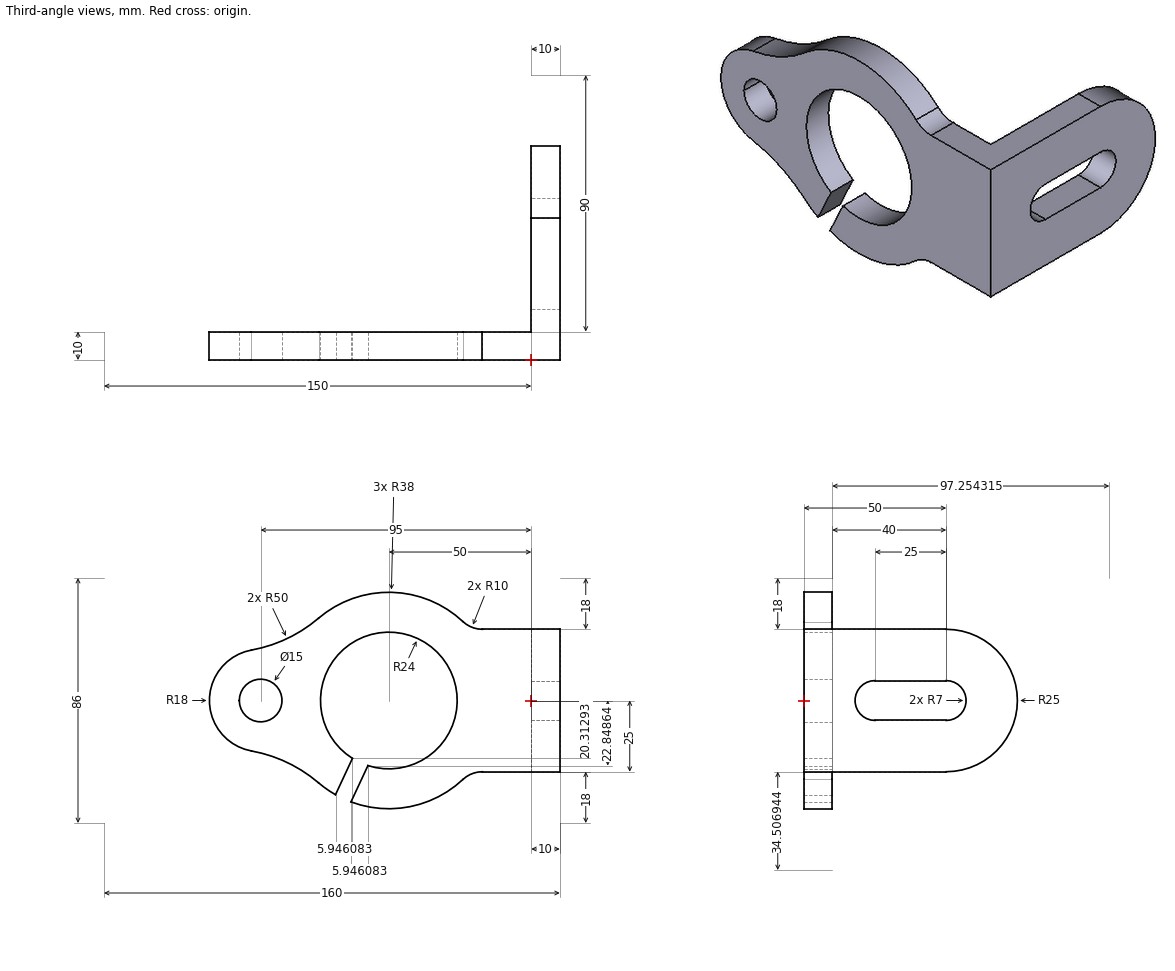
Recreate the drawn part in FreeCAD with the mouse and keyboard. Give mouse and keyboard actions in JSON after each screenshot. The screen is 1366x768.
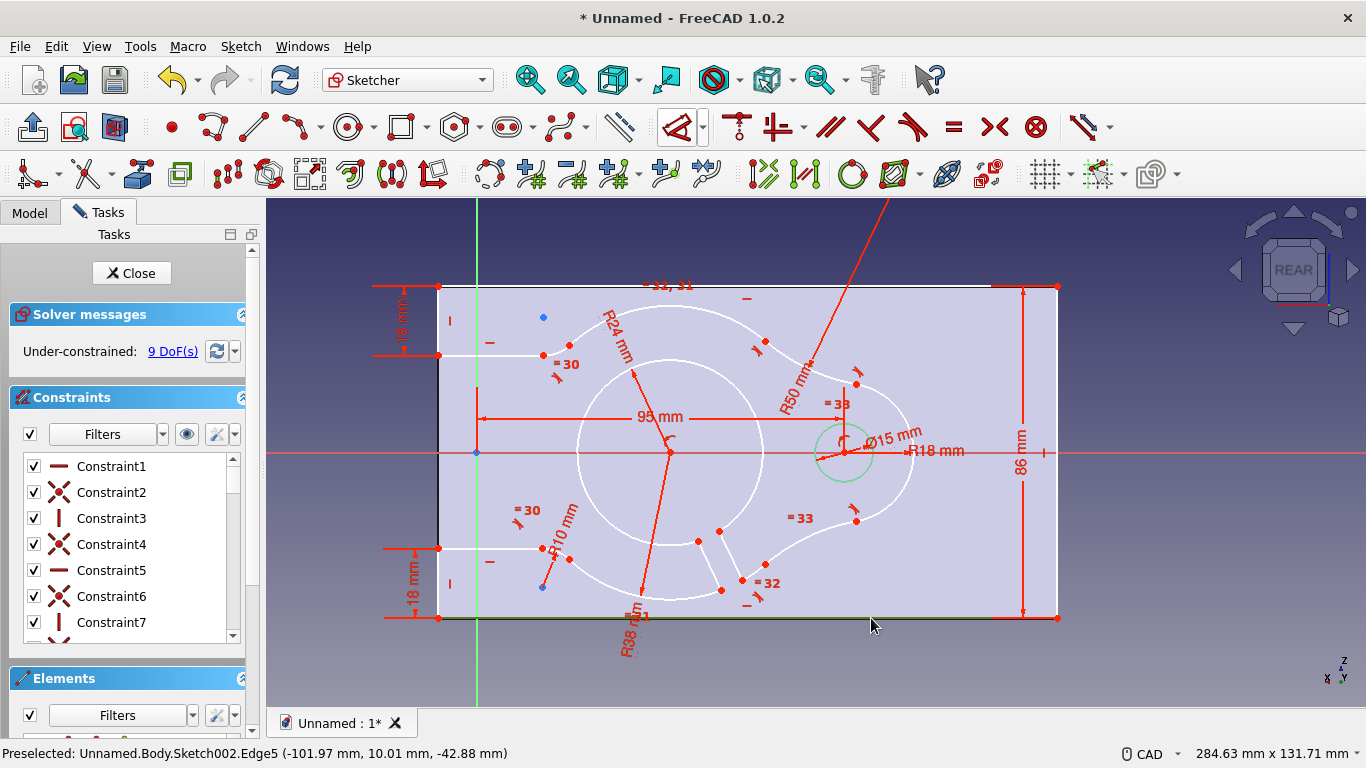
{"action": "key", "text": "l"}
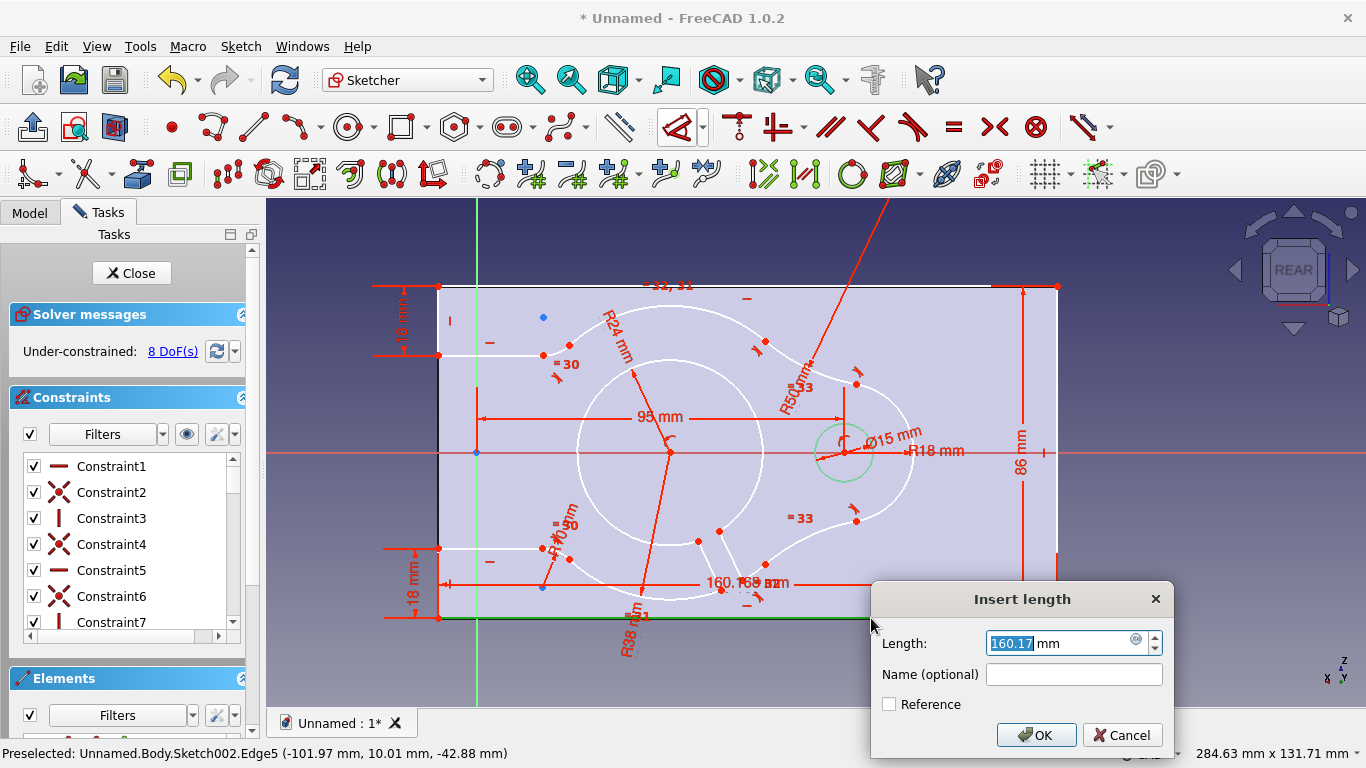
{"action": "type", "text": "160"}
{"action": "key", "text": "Return"}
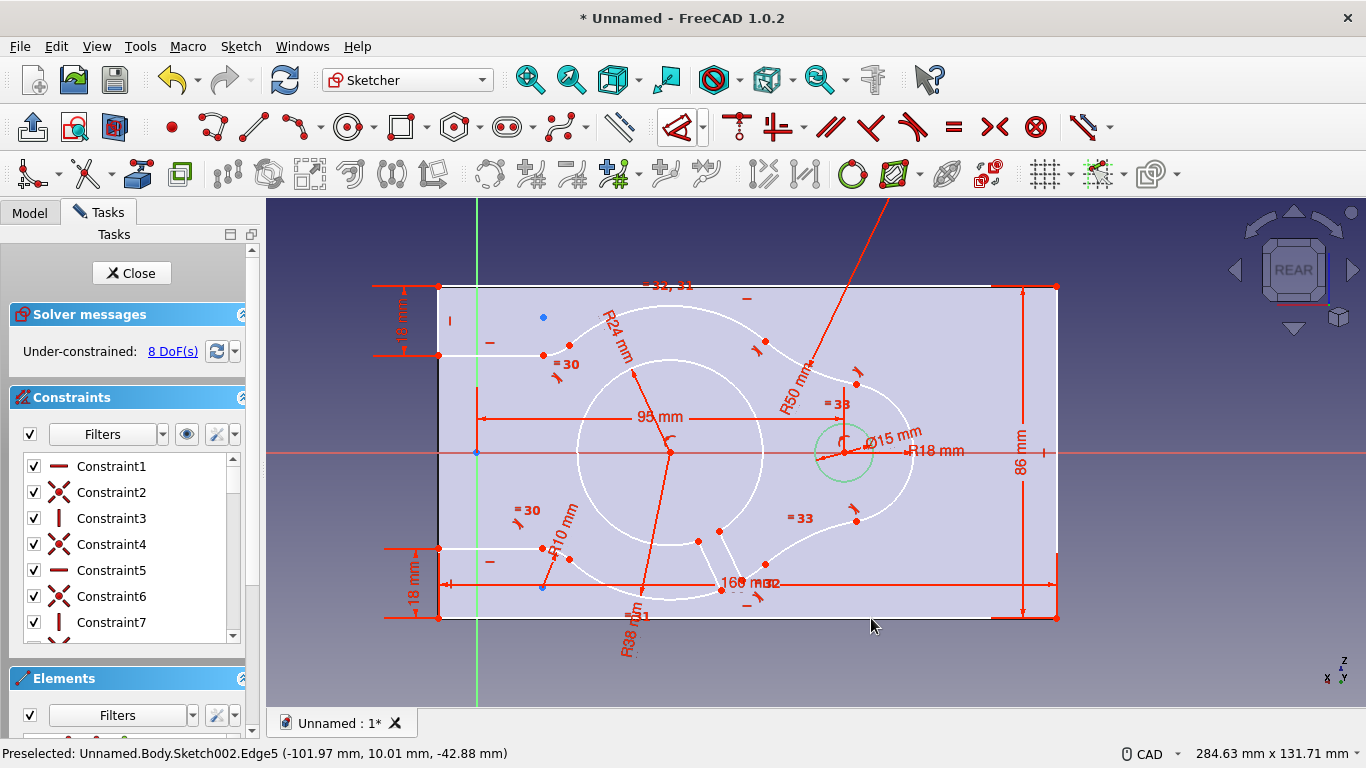
{"action": "left_click", "coordinate": [871, 286]}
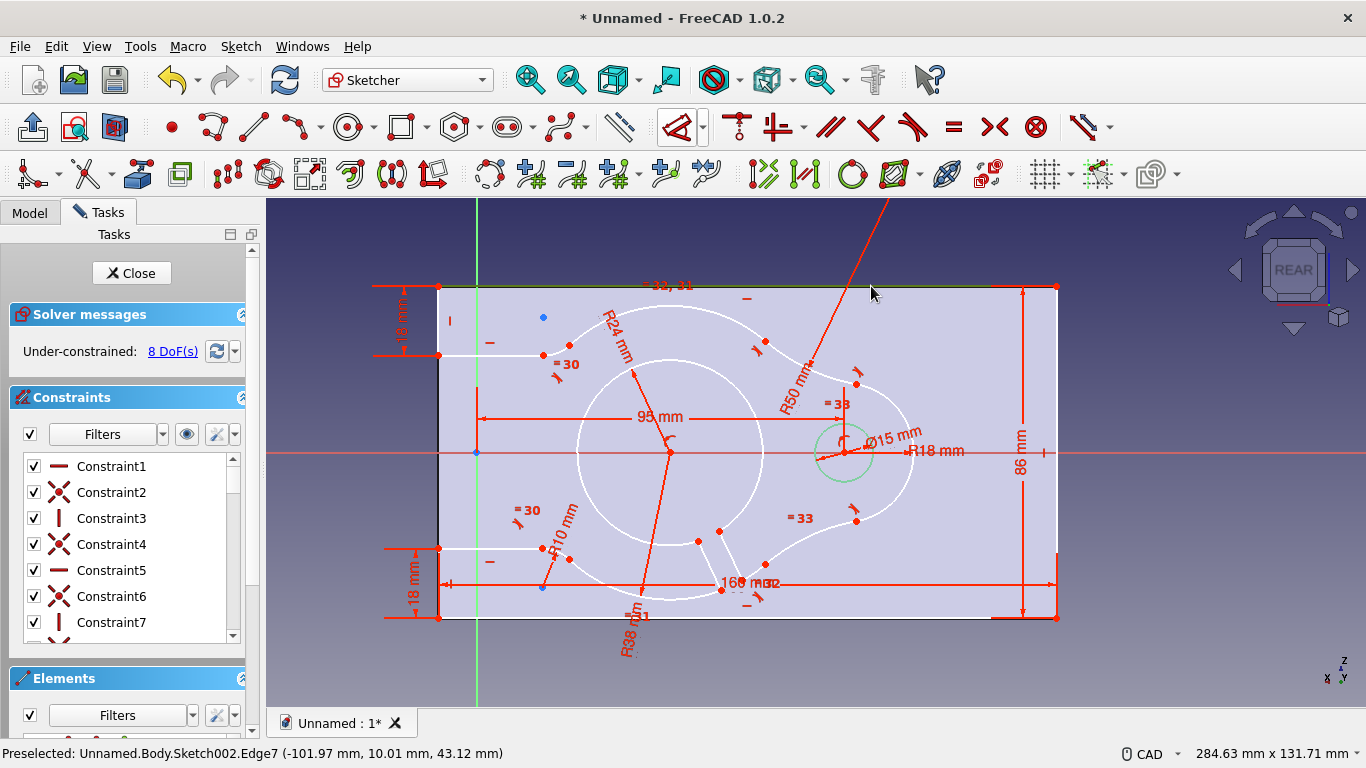
{"action": "key", "text": "l"}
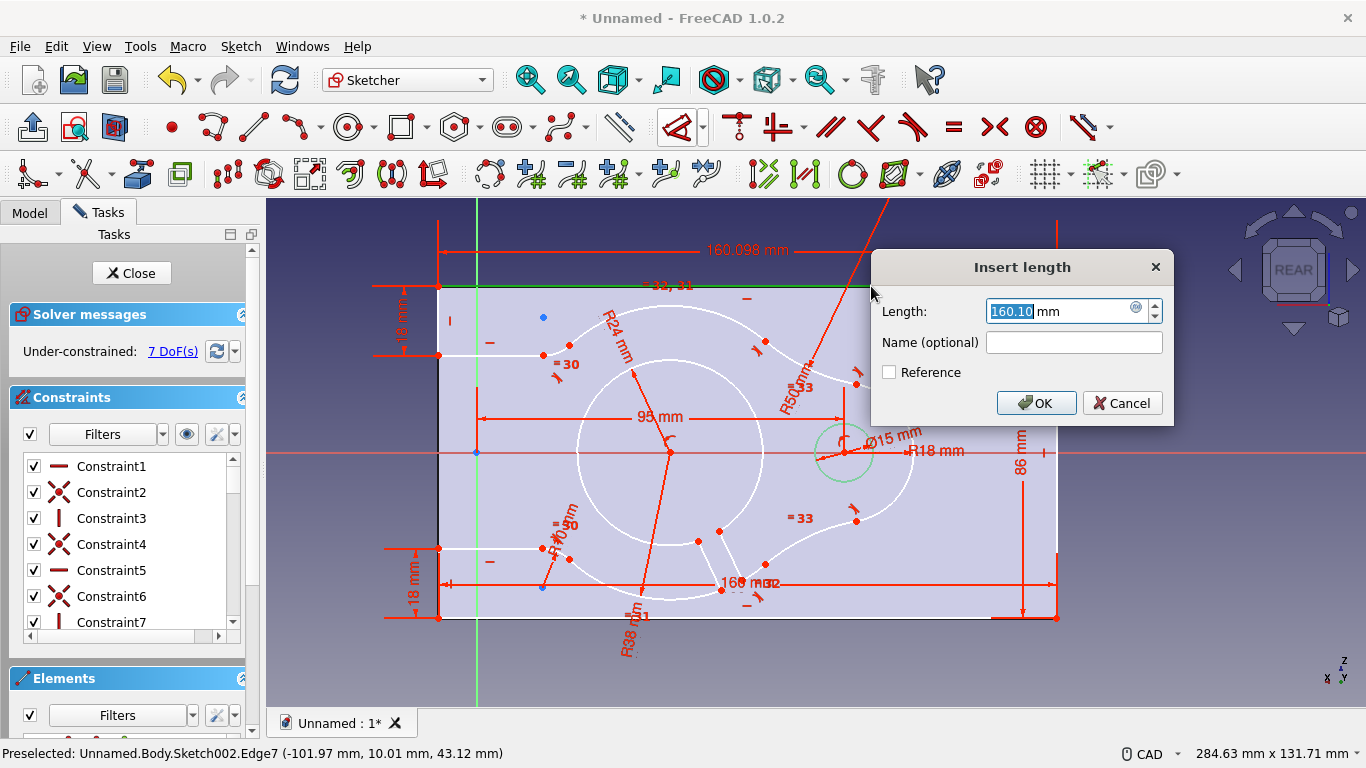
{"action": "type", "text": "160"}
{"action": "key", "text": "Return"}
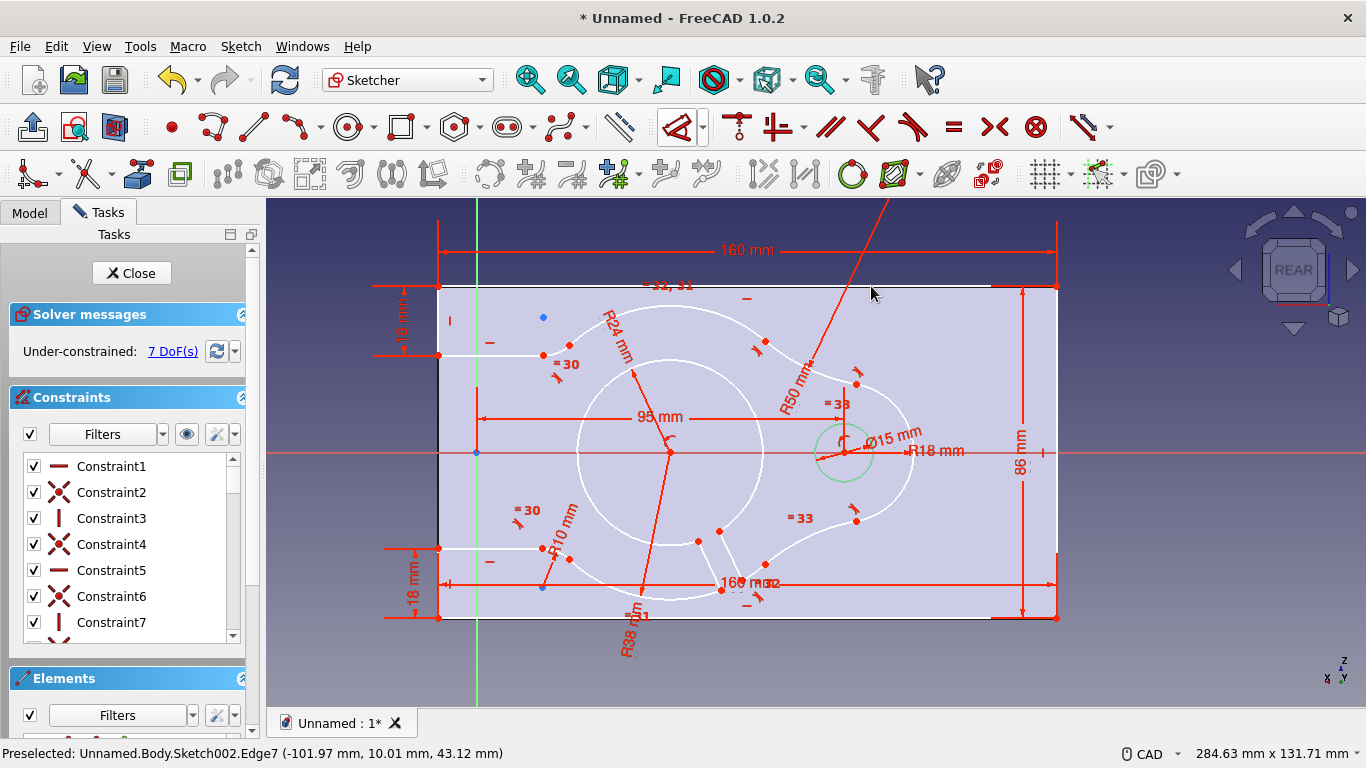
{"action": "left_click", "coordinate": [543, 549]}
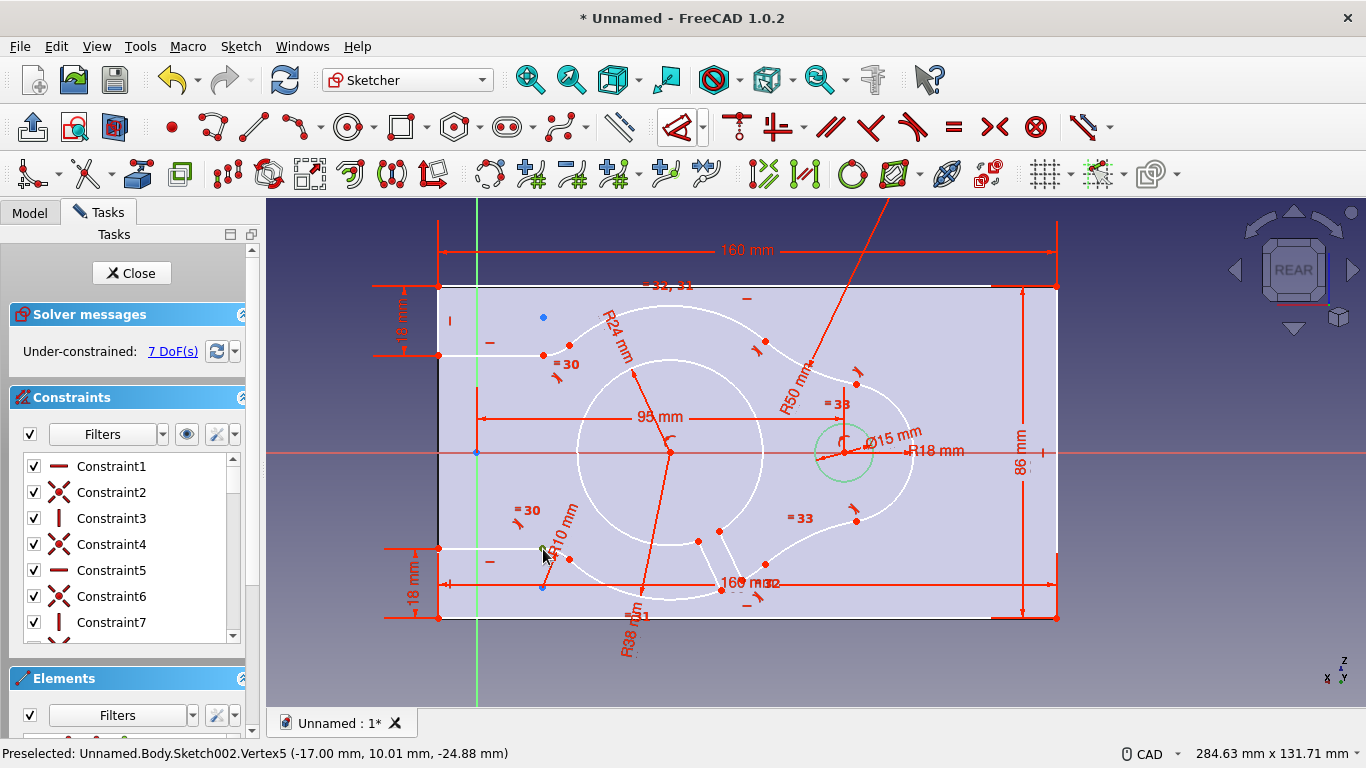
{"action": "key", "text": "i"}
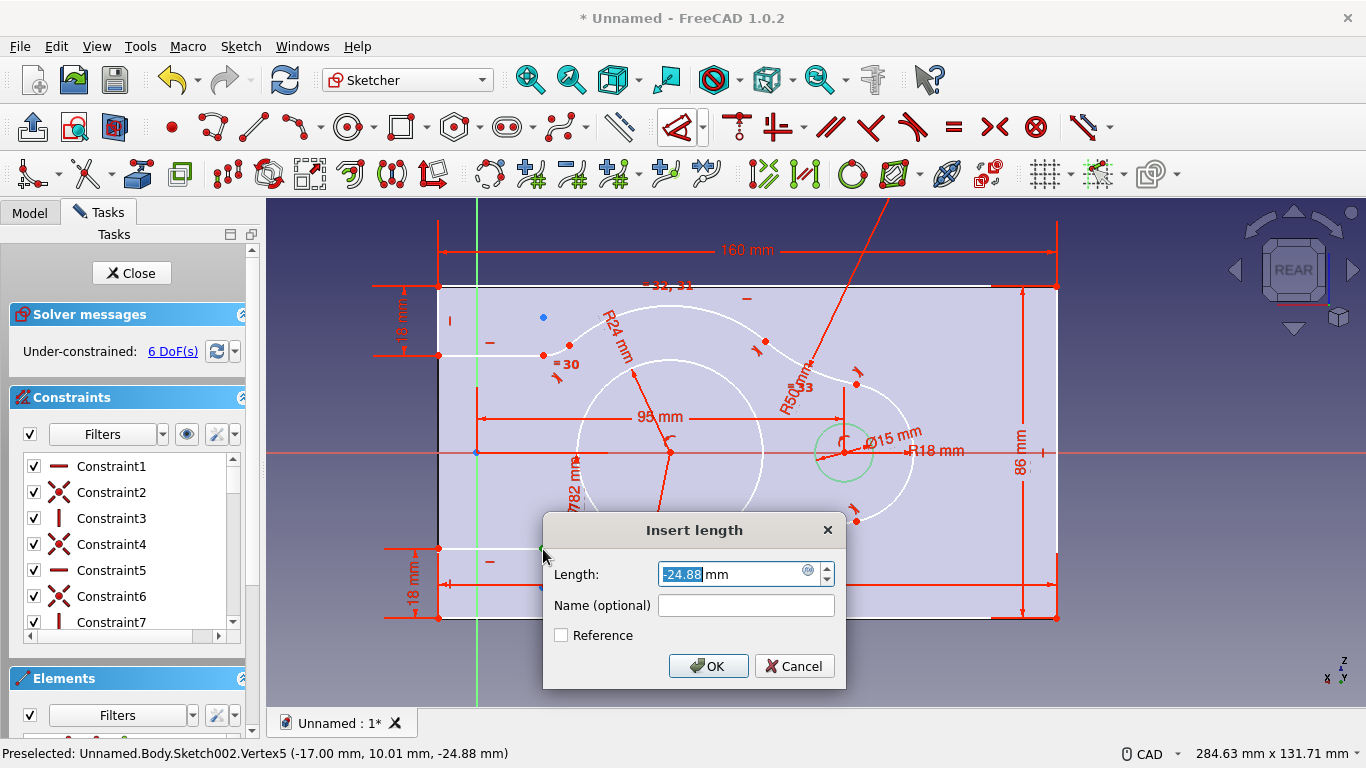
{"action": "type", "text": "-25"}
{"action": "key", "text": "Return"}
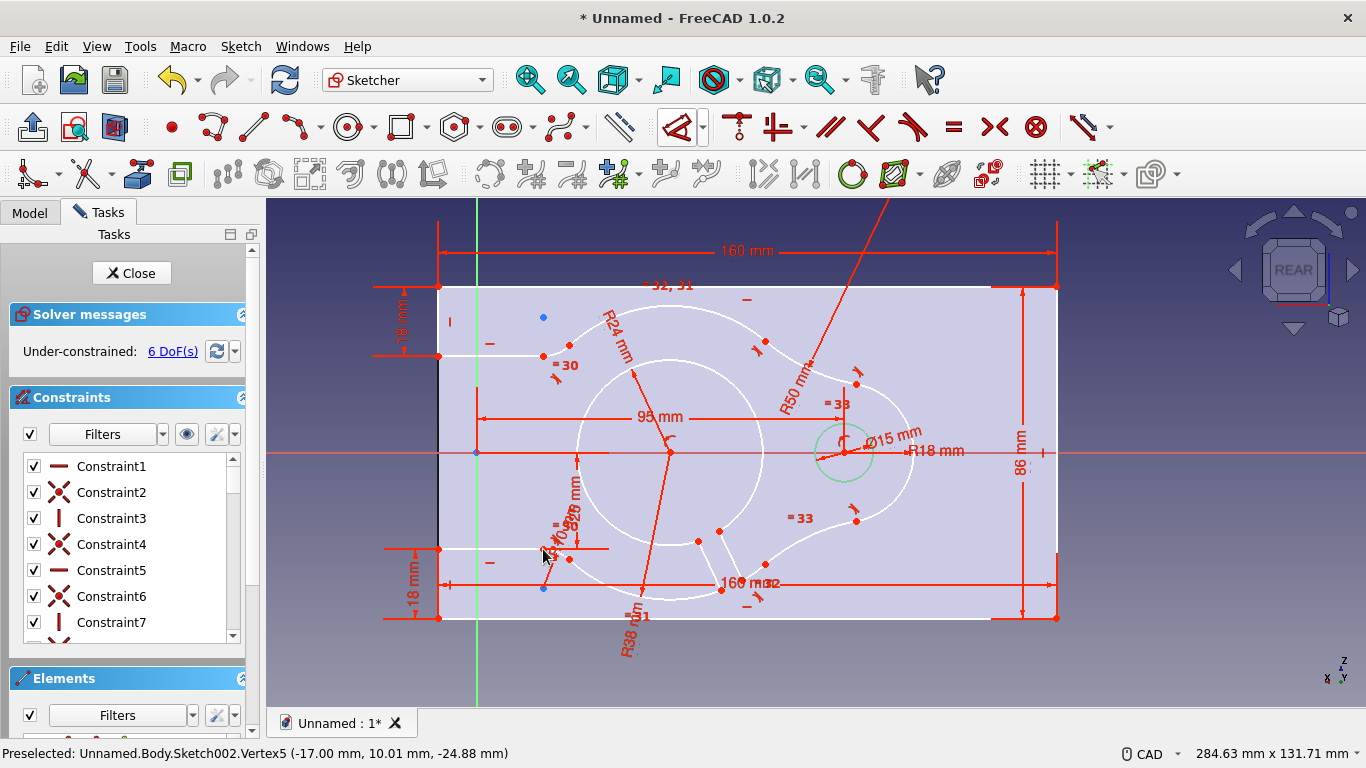
{"action": "left_click", "coordinate": [438, 549]}